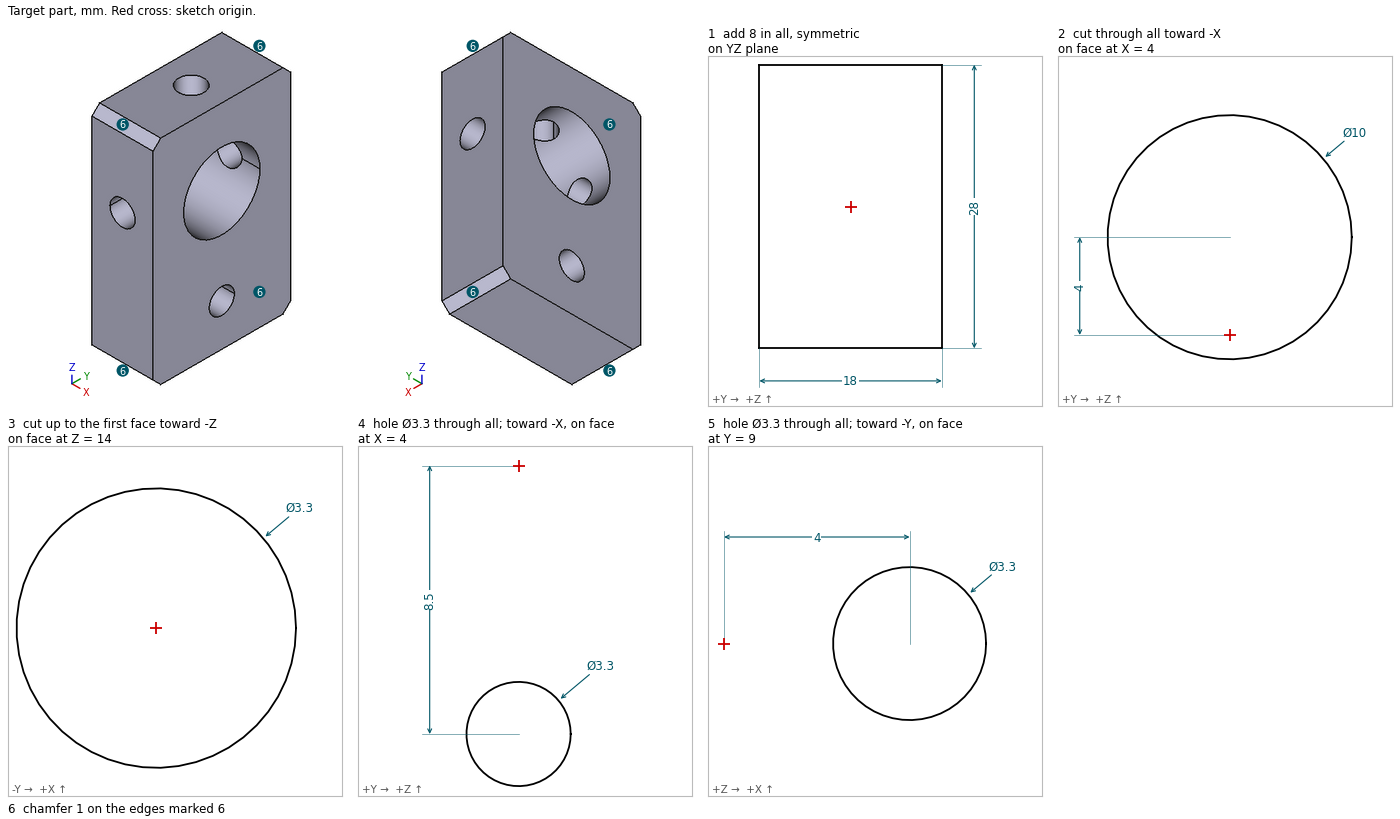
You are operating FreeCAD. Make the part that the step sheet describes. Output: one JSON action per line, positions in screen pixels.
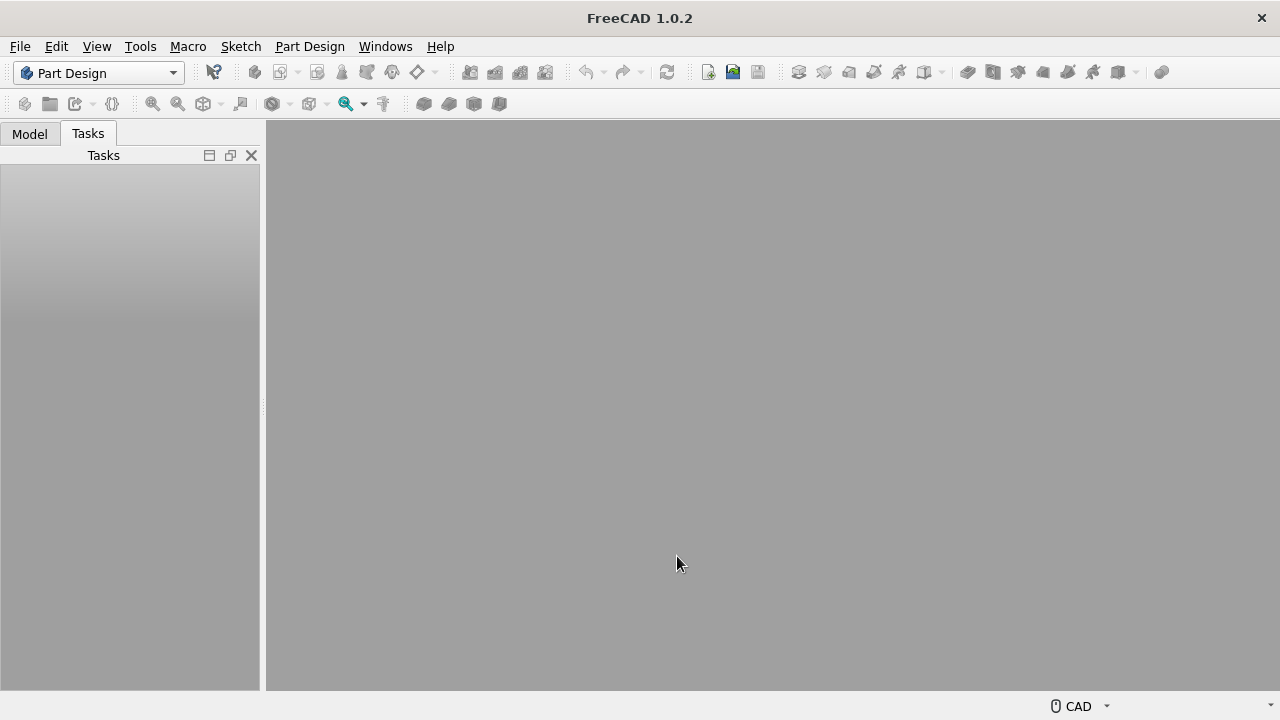
{"action": "left_click", "coordinate": [708, 72]}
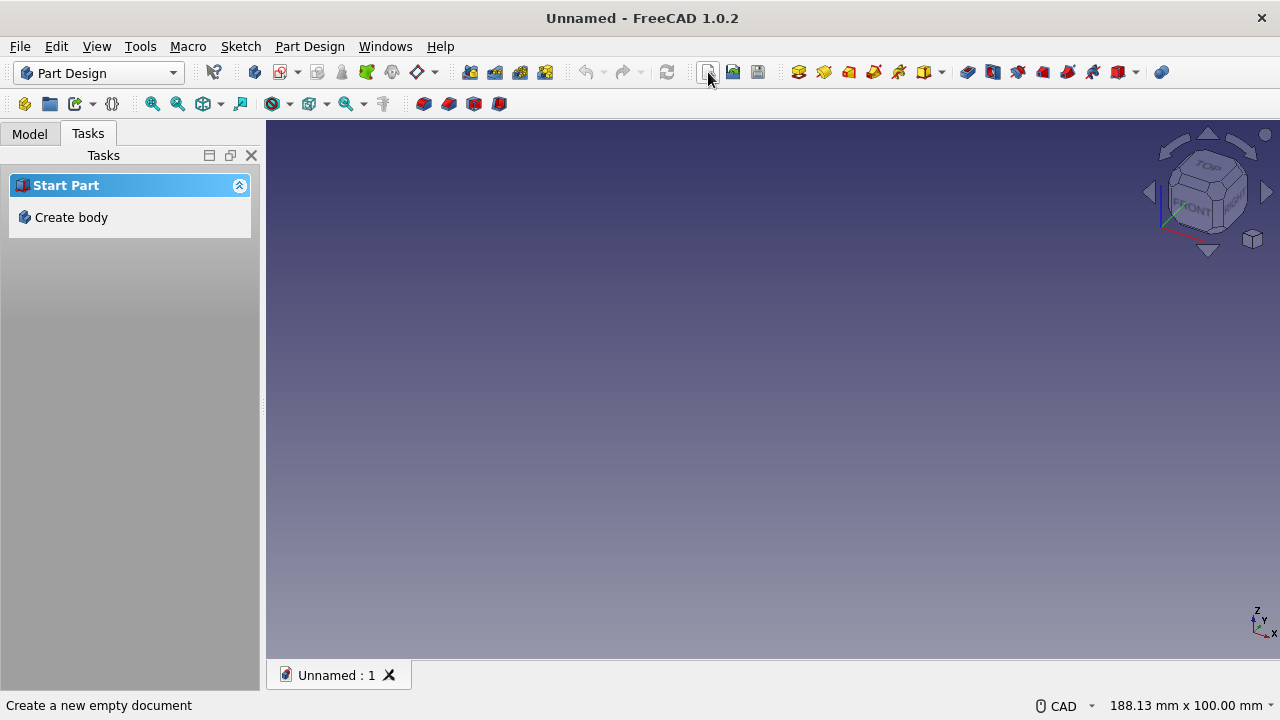
{"action": "left_click", "coordinate": [280, 72]}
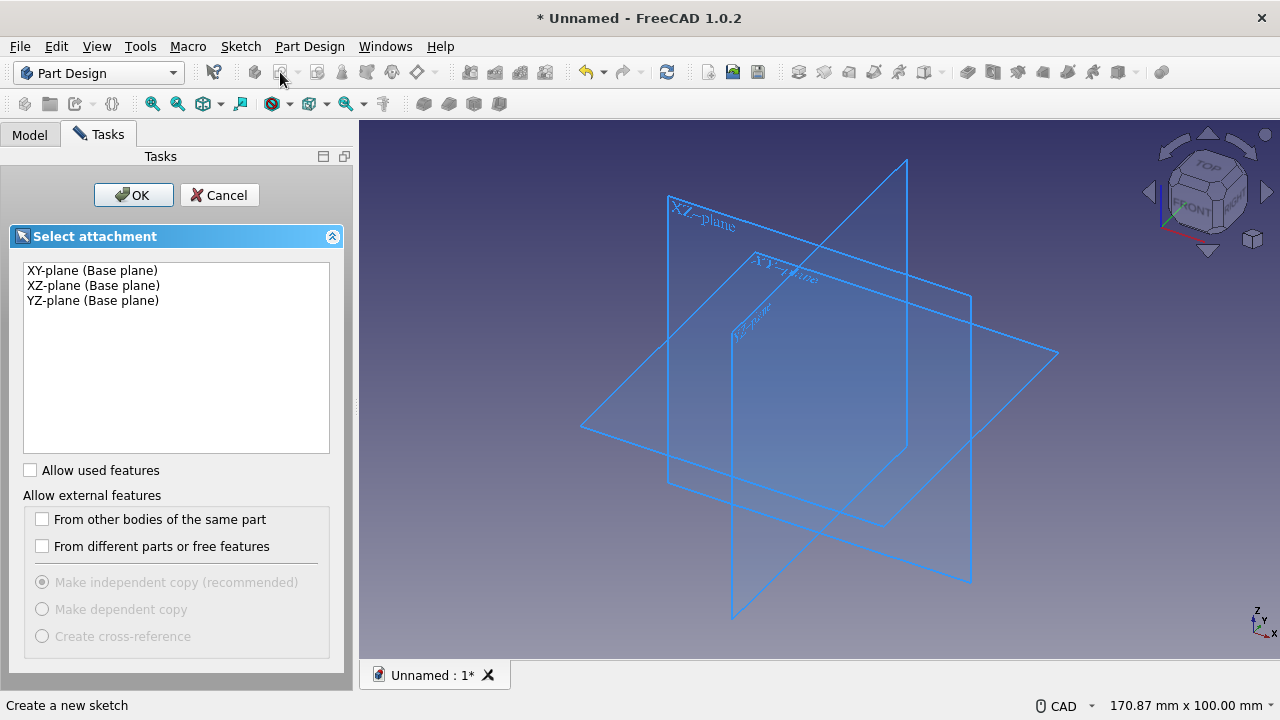
{"action": "left_click", "coordinate": [84, 300]}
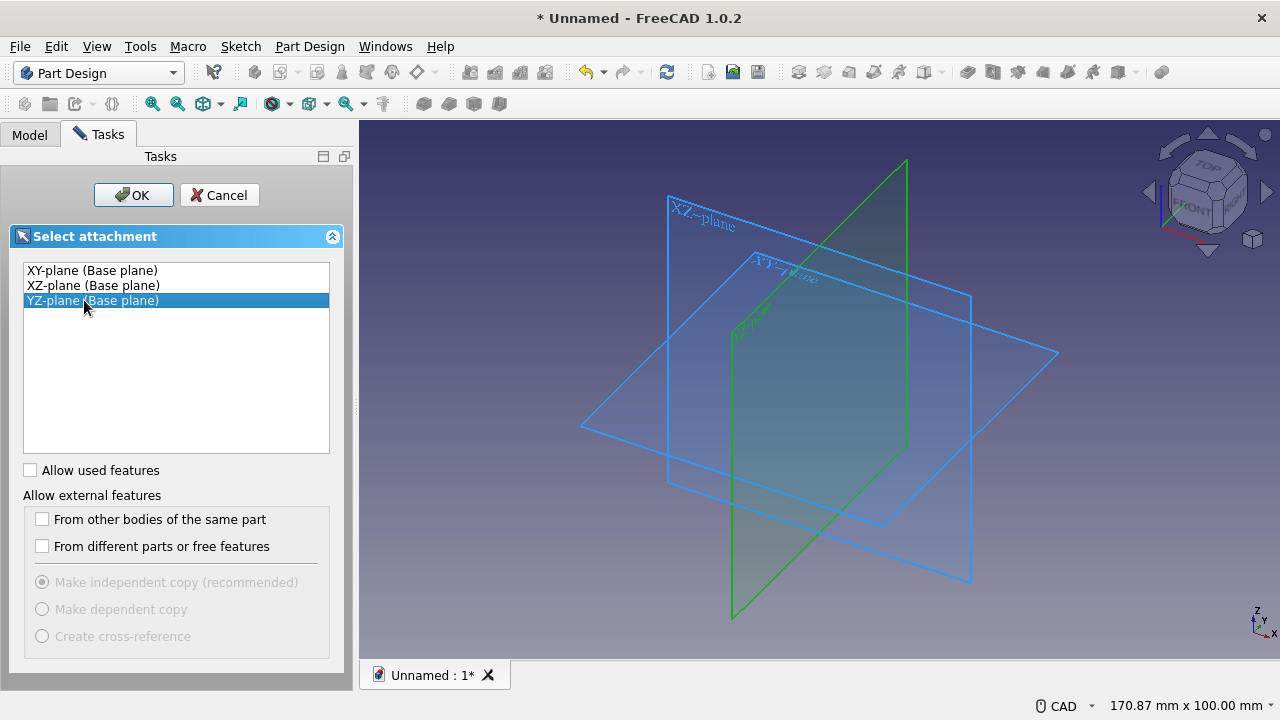
{"action": "left_click", "coordinate": [134, 195]}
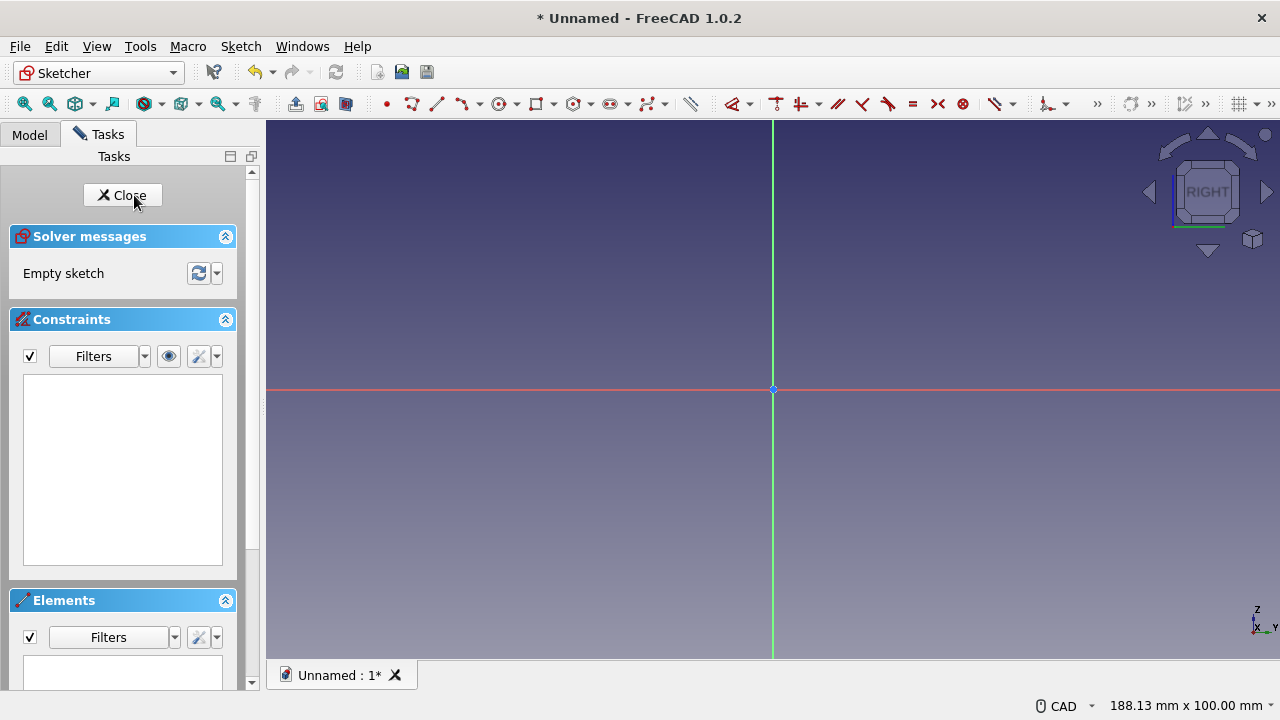
{"action": "scroll", "coordinate": [829, 390], "scroll_direction": "up", "scroll_amount": 4}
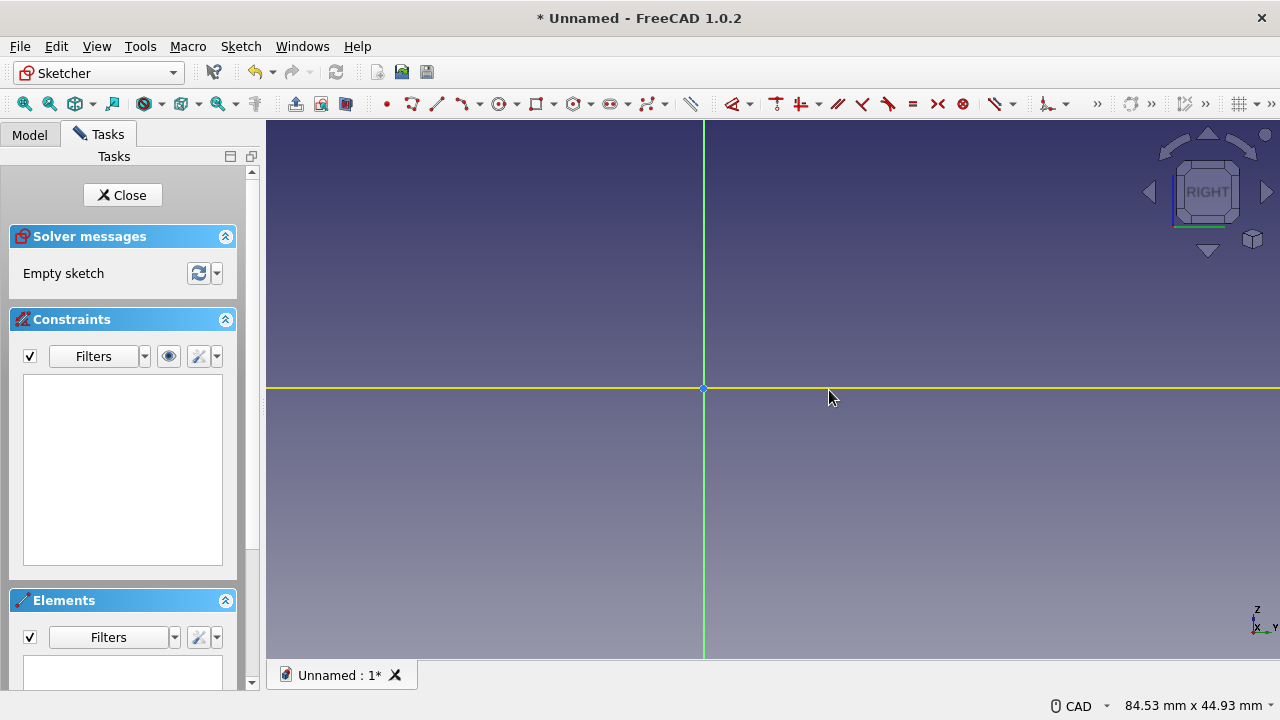
{"action": "left_click", "coordinate": [554, 104]}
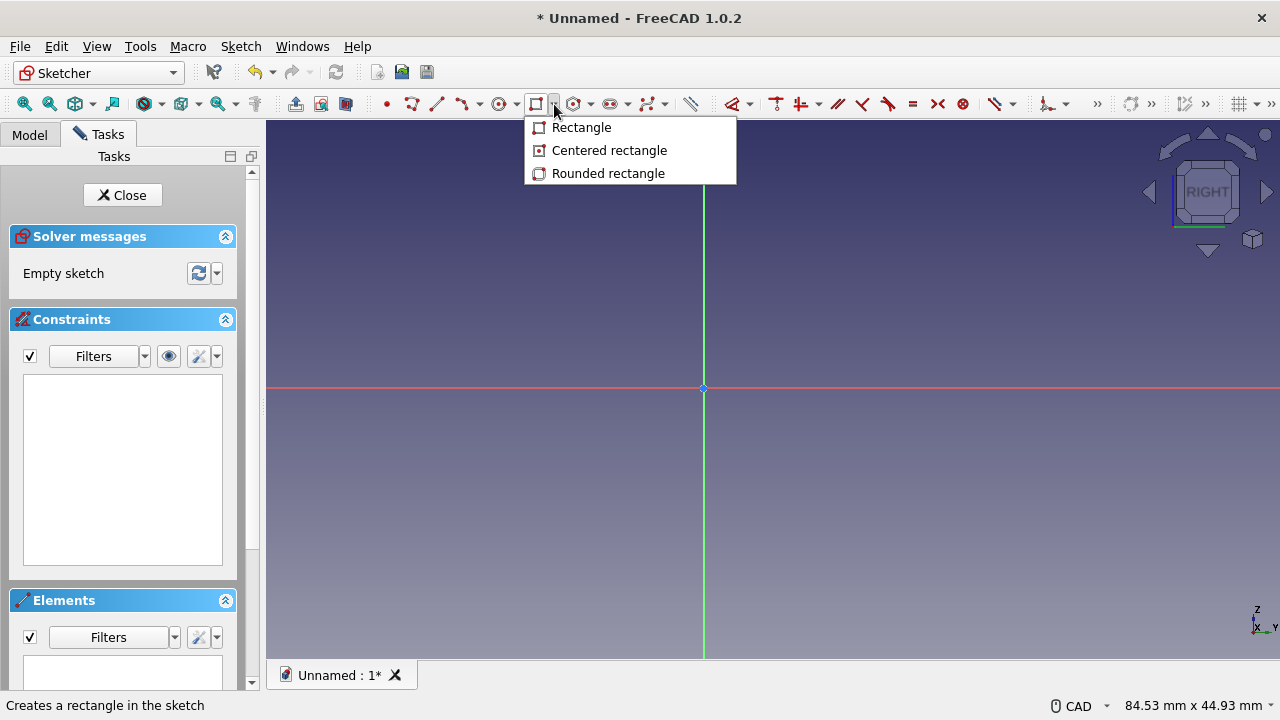
{"action": "left_click", "coordinate": [630, 150]}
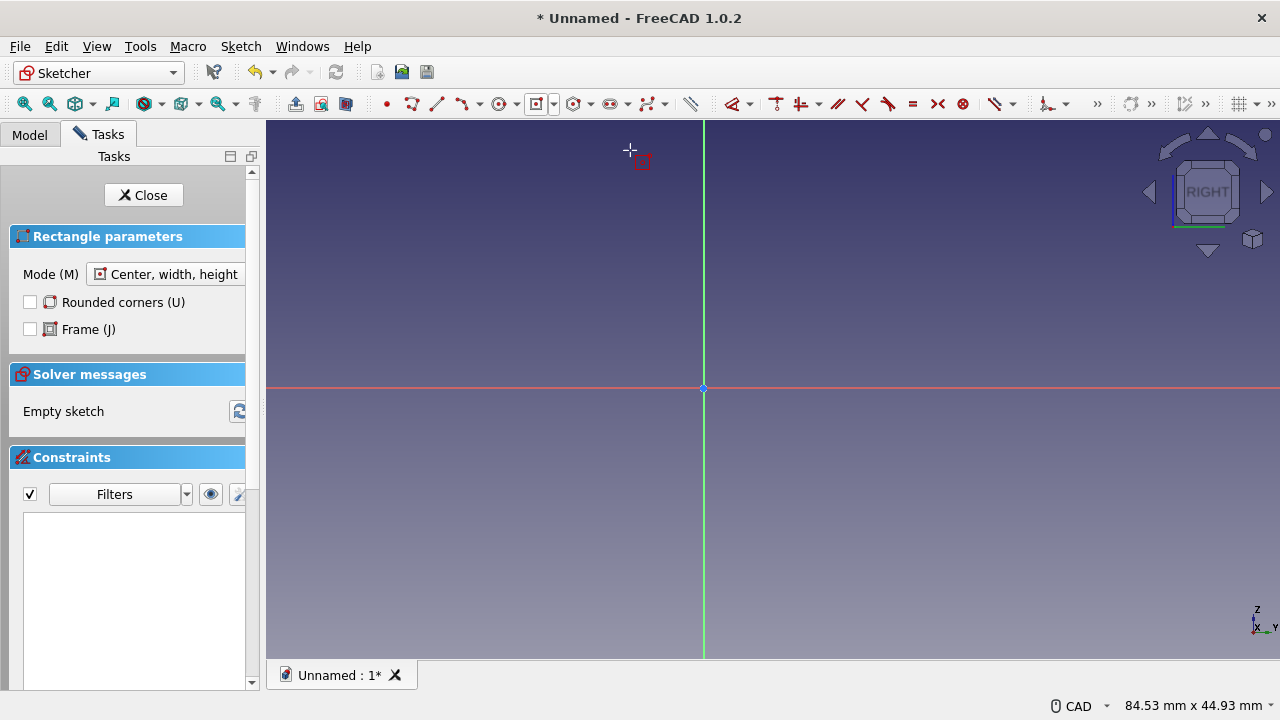
{"action": "left_click", "coordinate": [704, 388]}
{"action": "left_click", "coordinate": [812, 220]}
{"action": "key", "text": "Escape"}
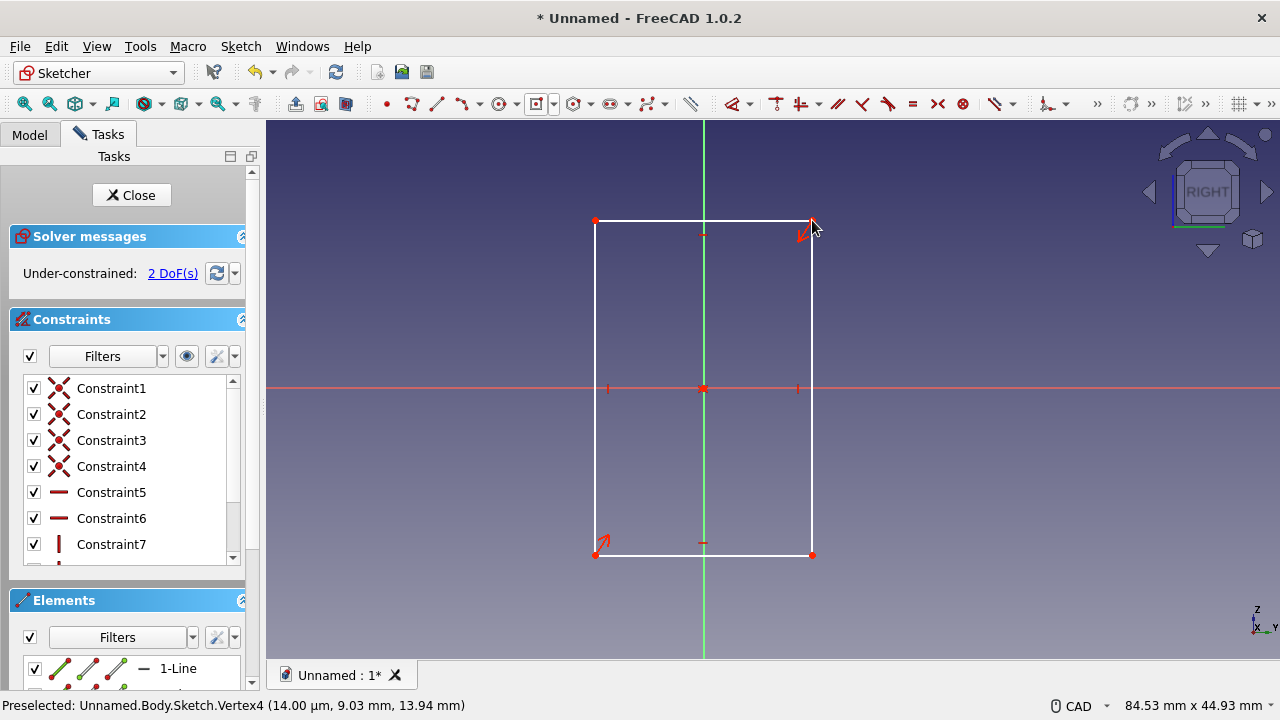
{"action": "left_click", "coordinate": [660, 556]}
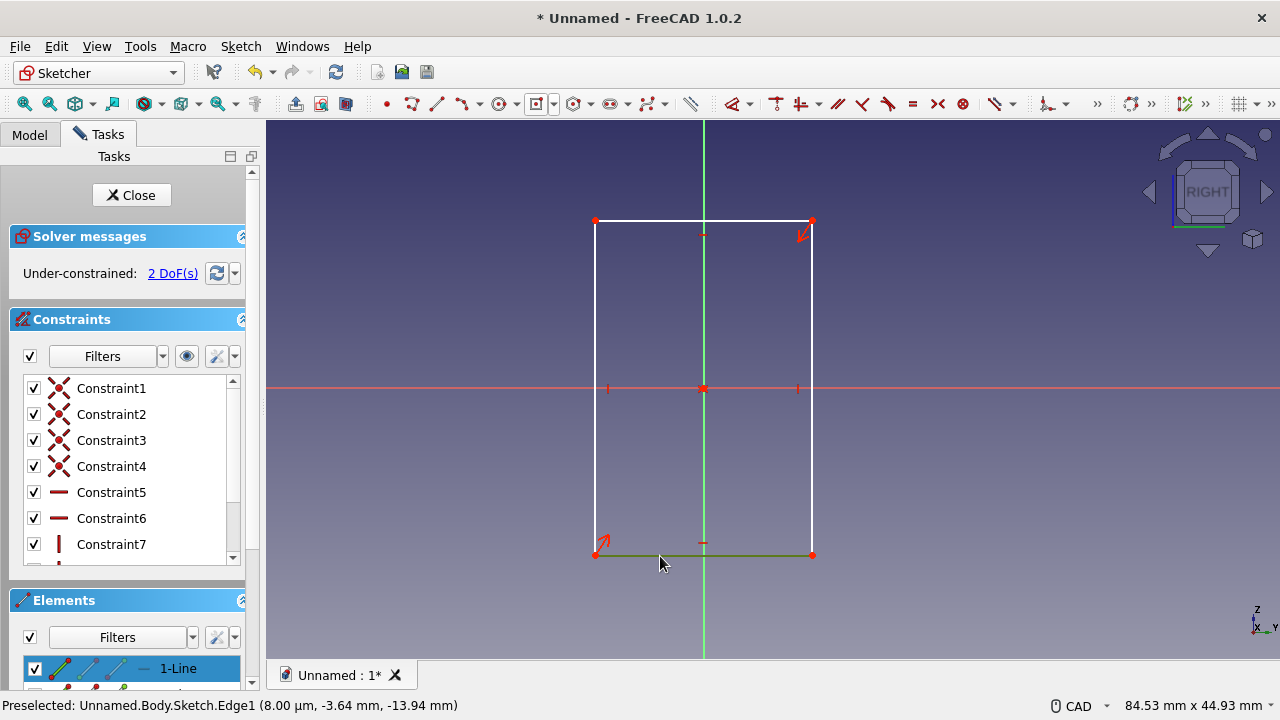
{"action": "key", "text": "l"}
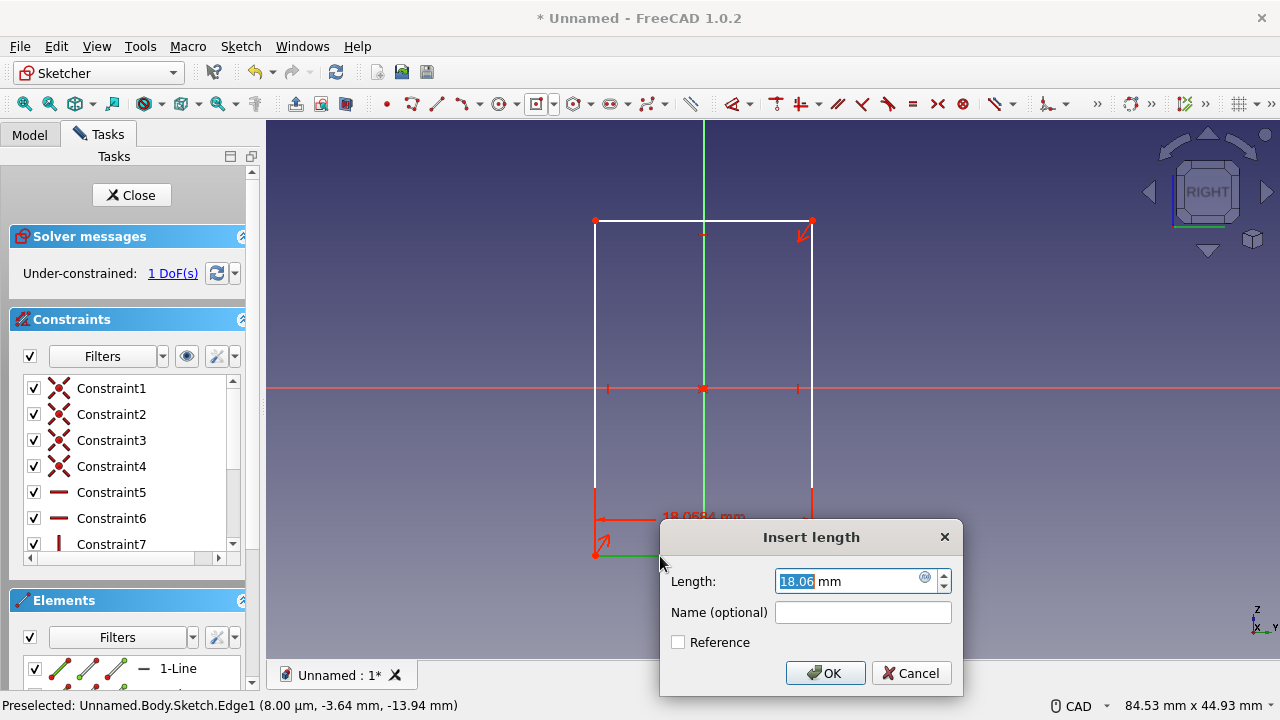
{"action": "type", "text": "18"}
{"action": "key", "text": "Return"}